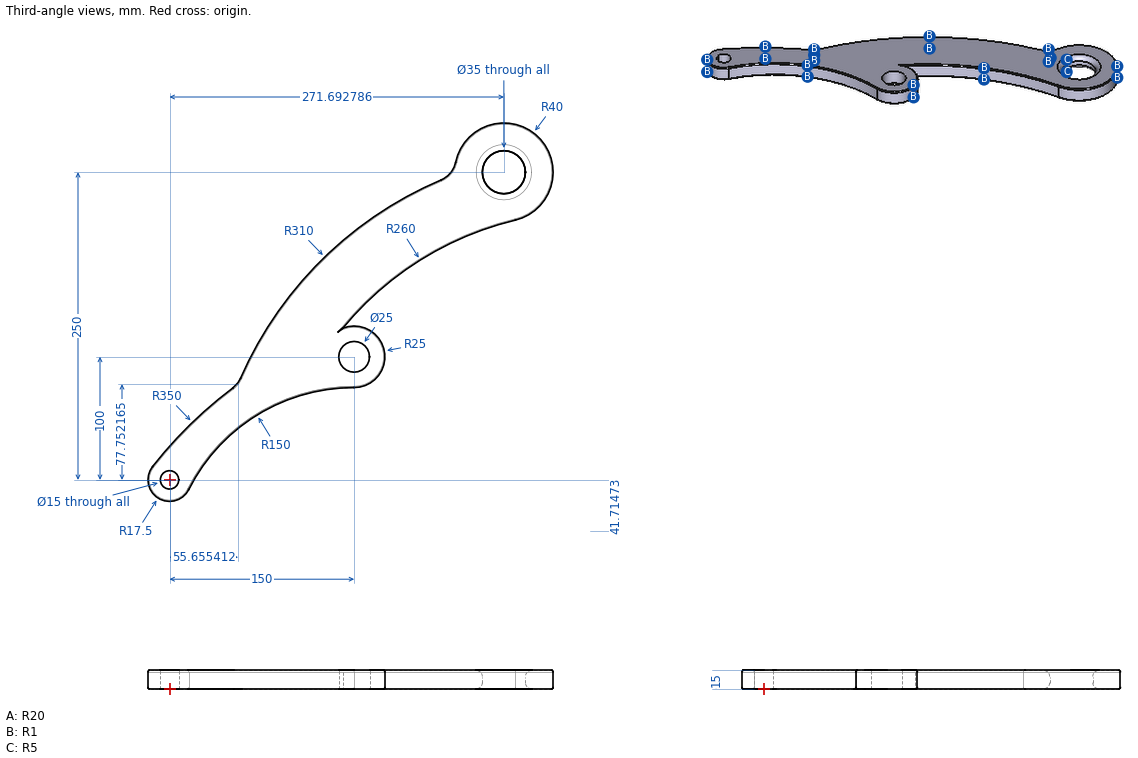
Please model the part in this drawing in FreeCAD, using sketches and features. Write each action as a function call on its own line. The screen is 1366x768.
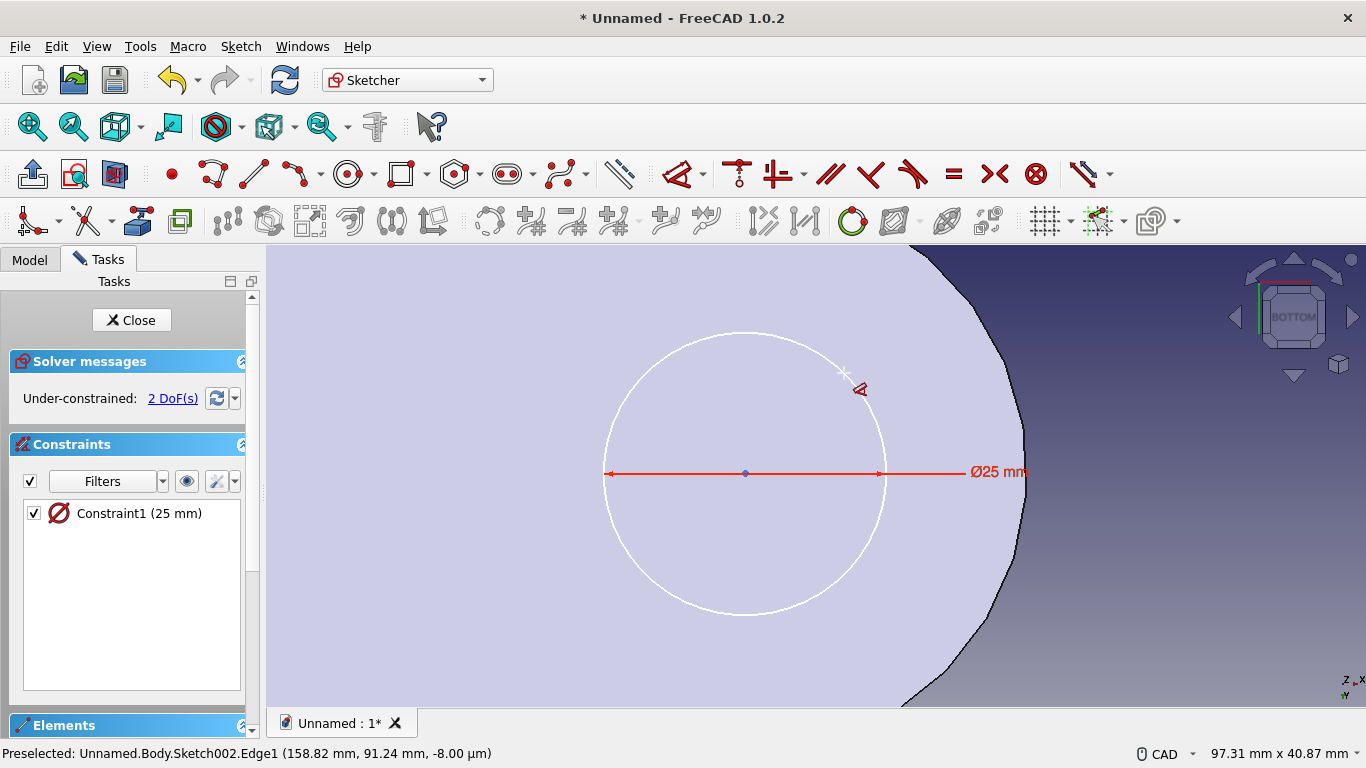
click(745, 474)
click(520, 508)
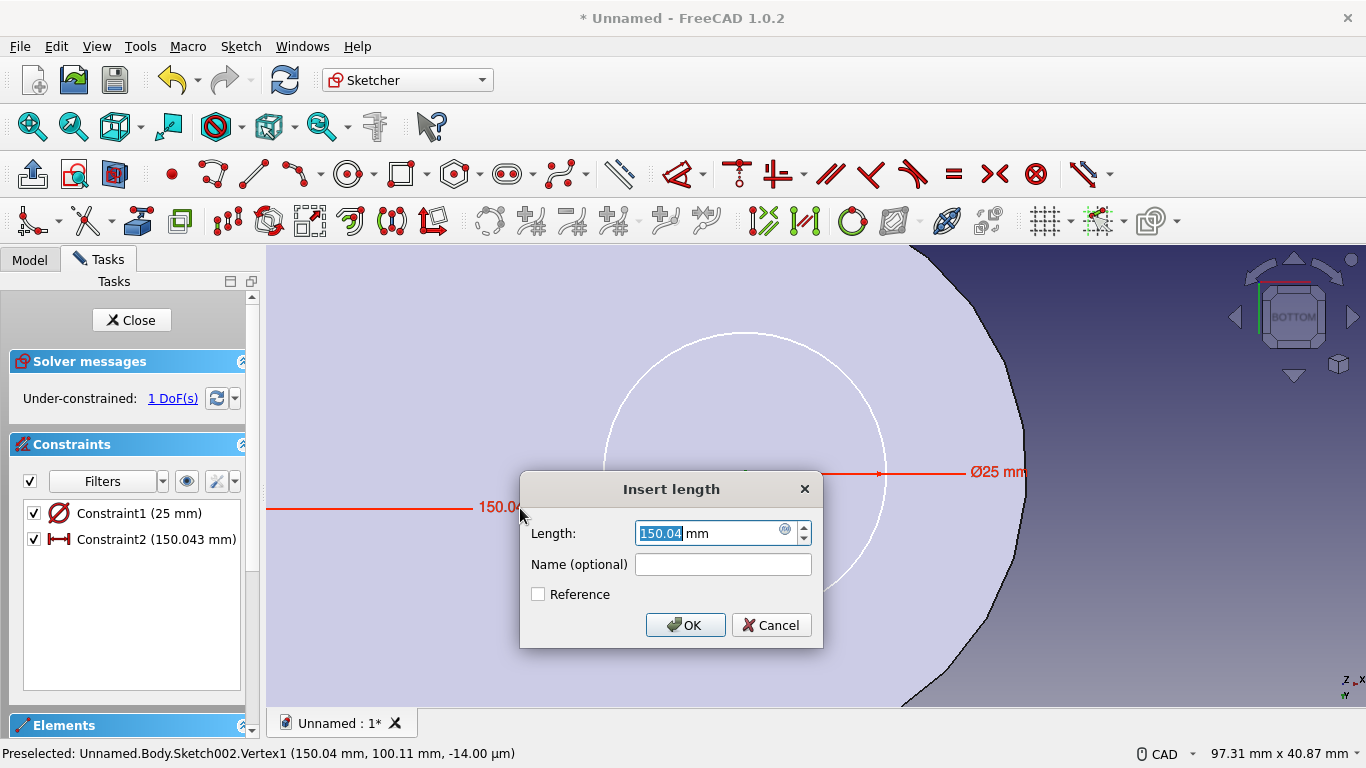
text(150)
key(Return)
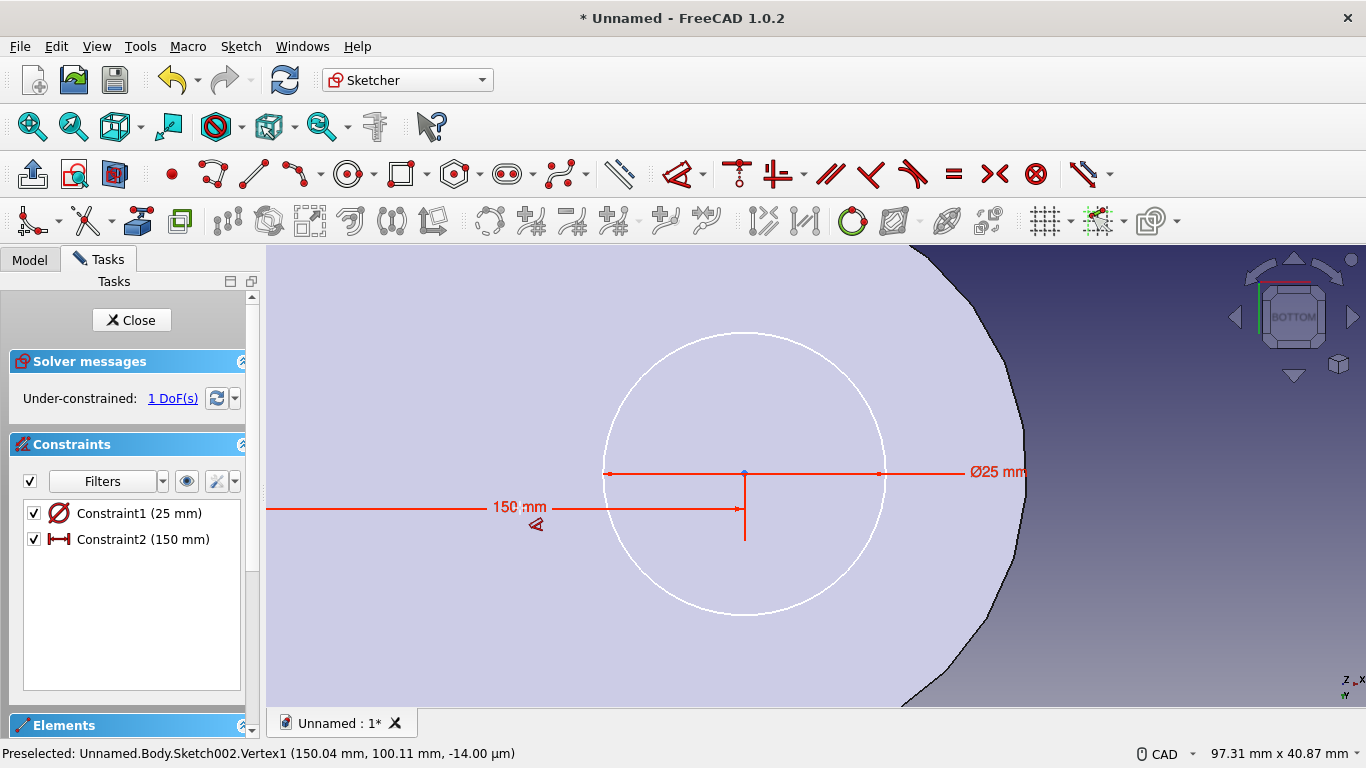
click(745, 474)
click(779, 374)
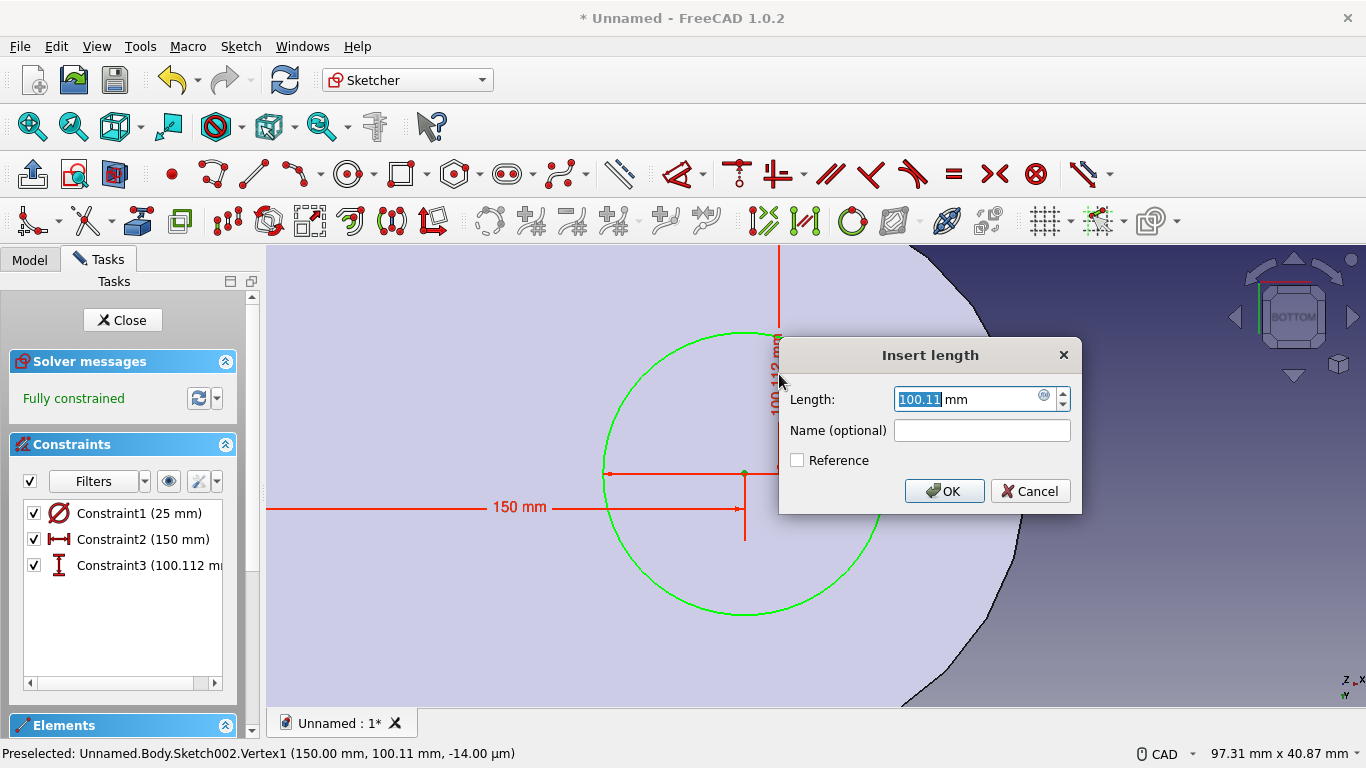
text(100)
key(Return)
key(Escape)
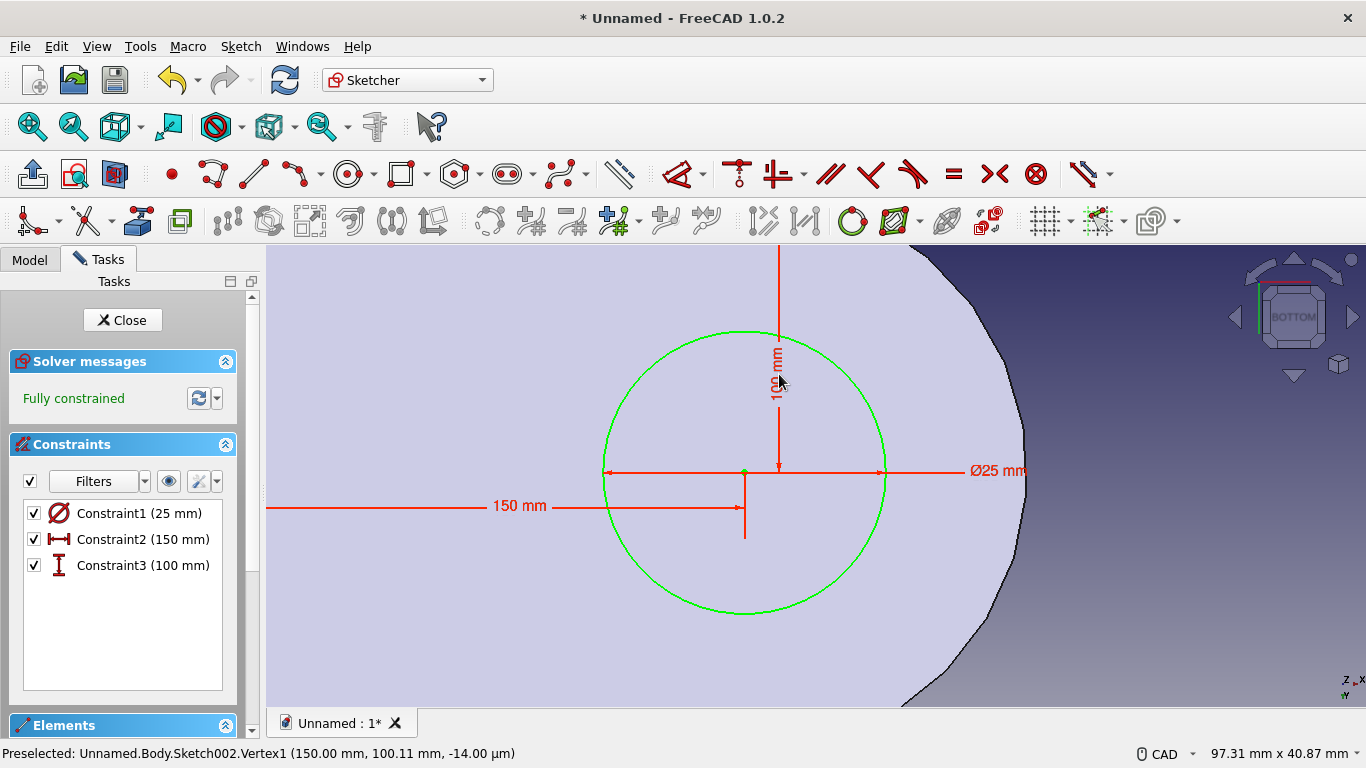
click(123, 320)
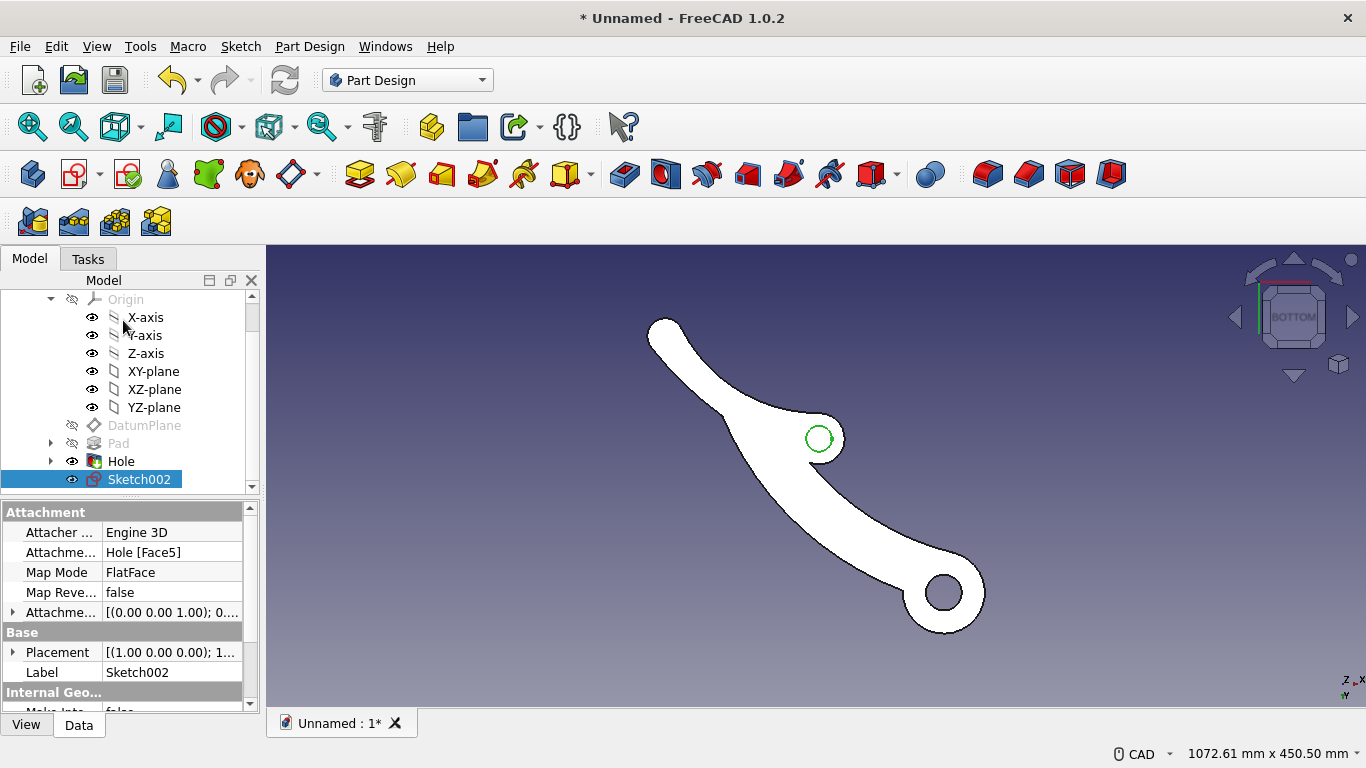
click(625, 174)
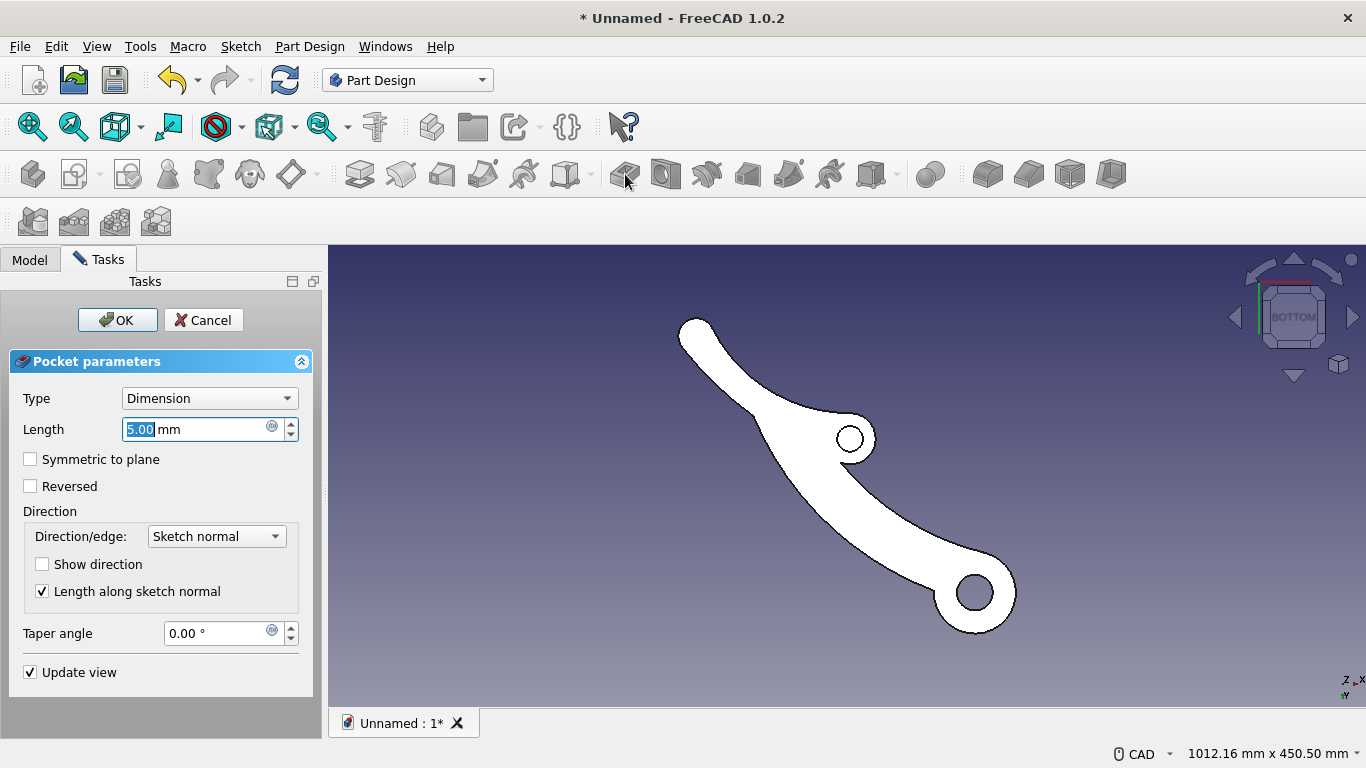
click(210, 398)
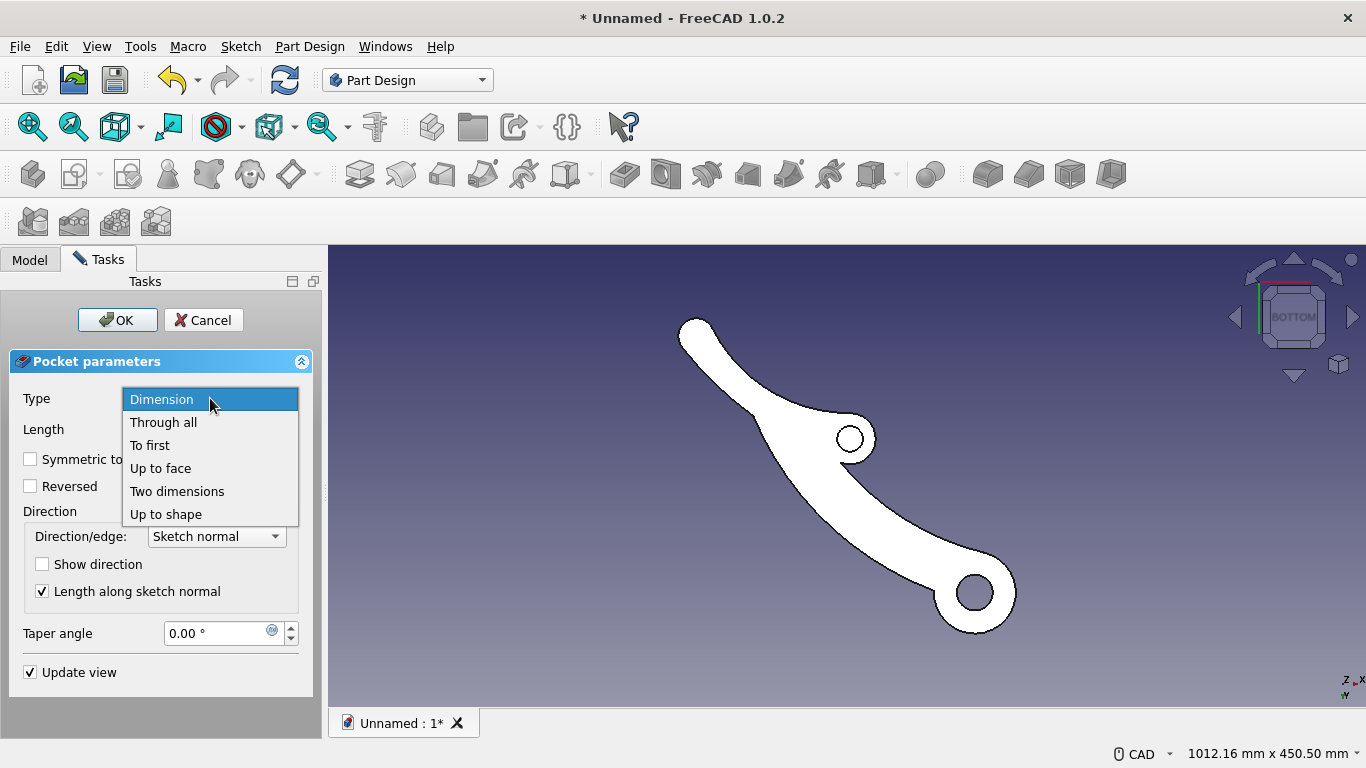
click(208, 422)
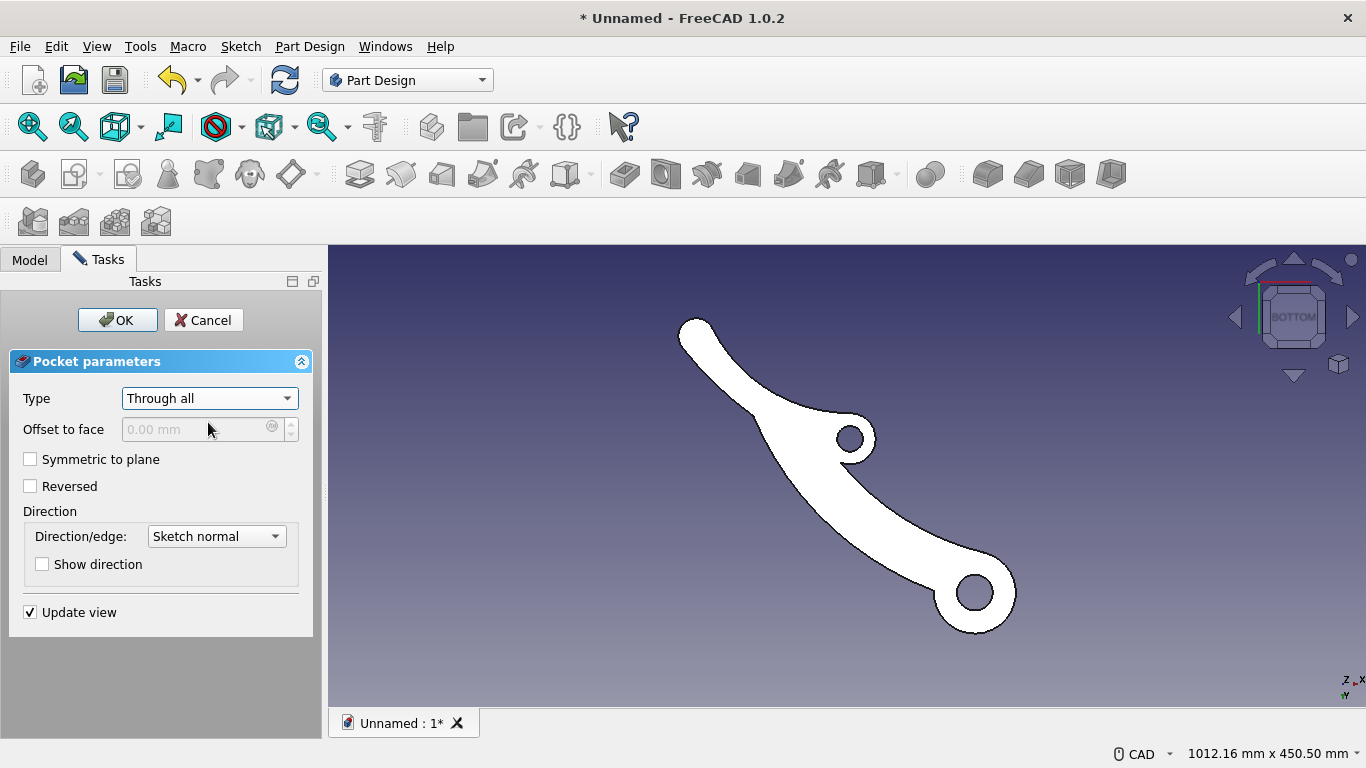
click(118, 320)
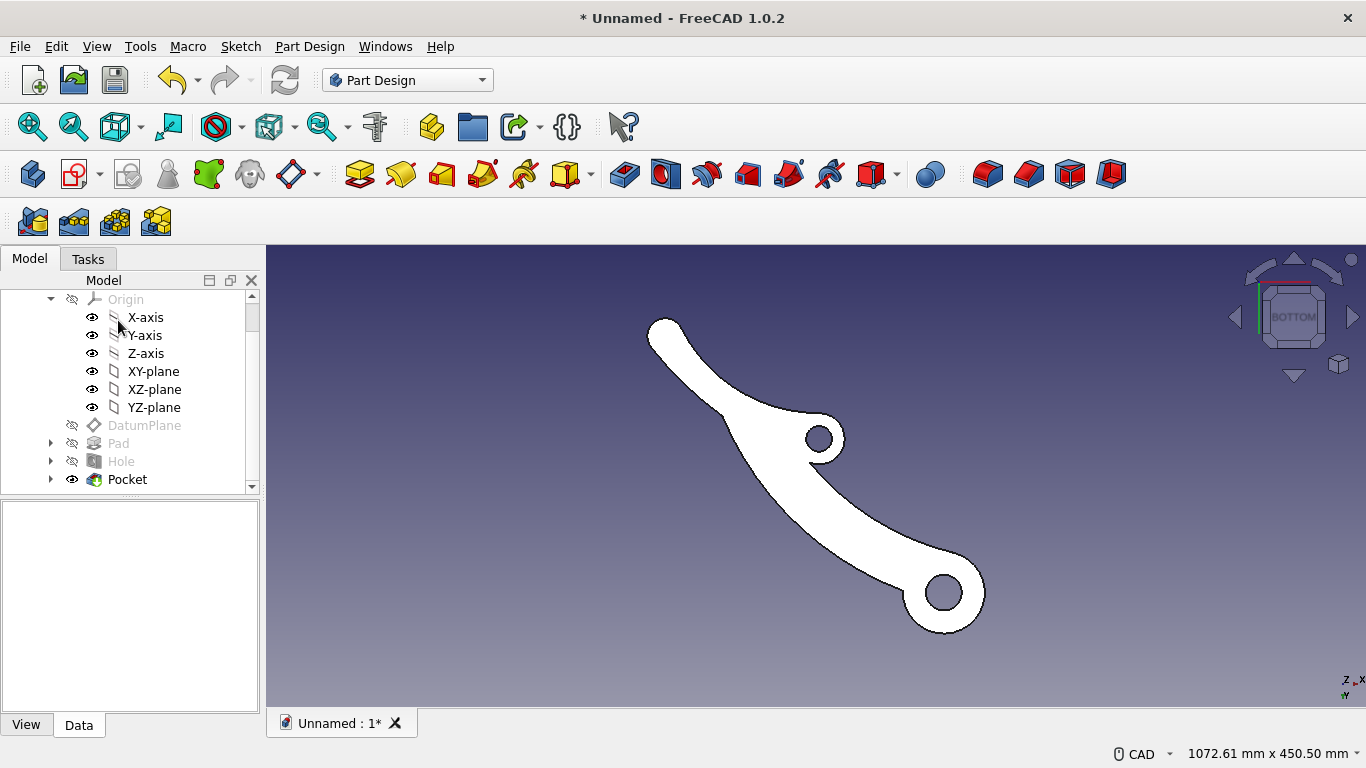
click(768, 430)